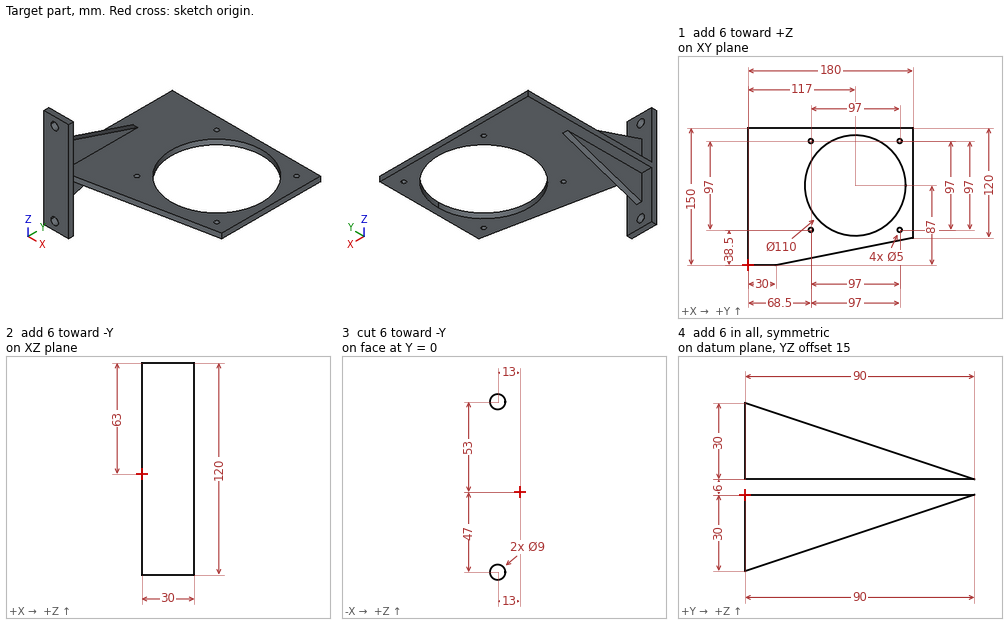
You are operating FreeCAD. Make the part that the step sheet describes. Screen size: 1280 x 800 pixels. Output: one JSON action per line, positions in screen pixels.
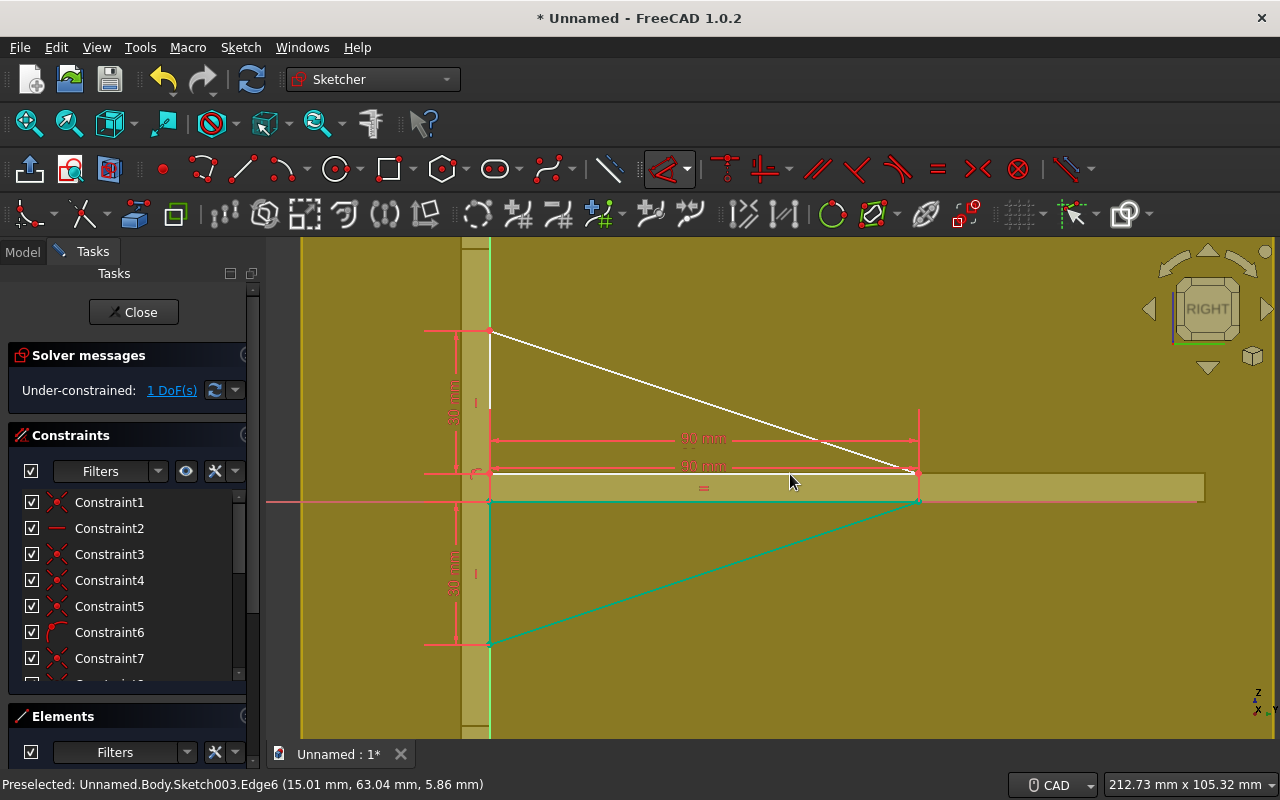
{"action": "scroll", "coordinate": [490, 474], "scroll_direction": "up", "scroll_amount": 2}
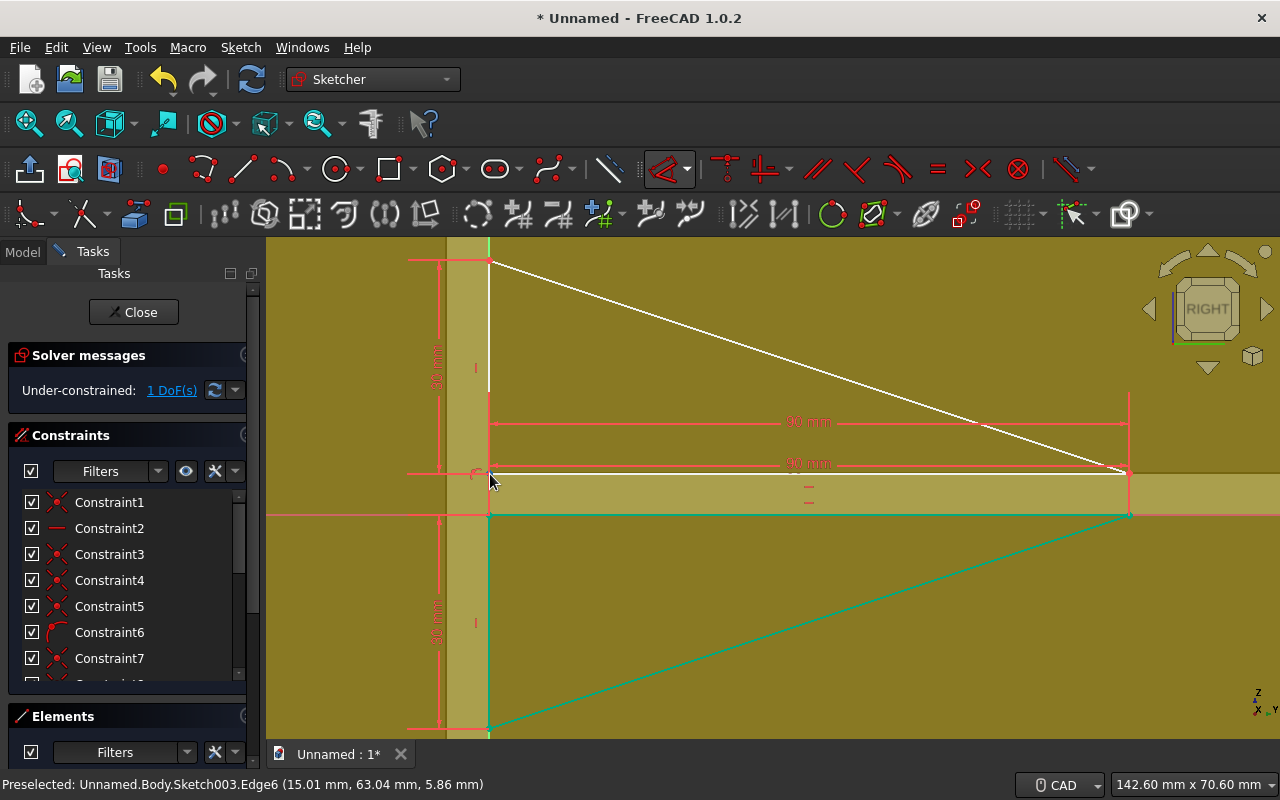
{"action": "left_click", "coordinate": [489, 474]}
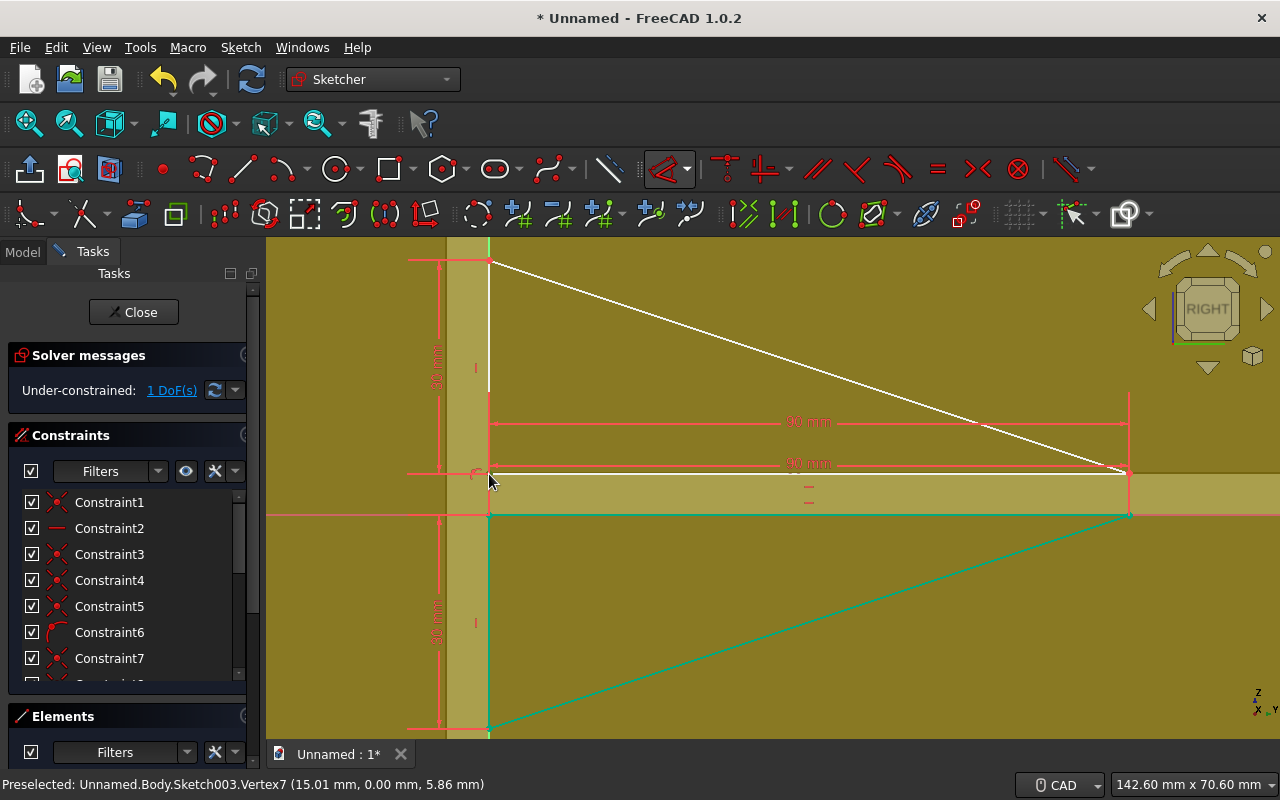
{"action": "key", "text": "i"}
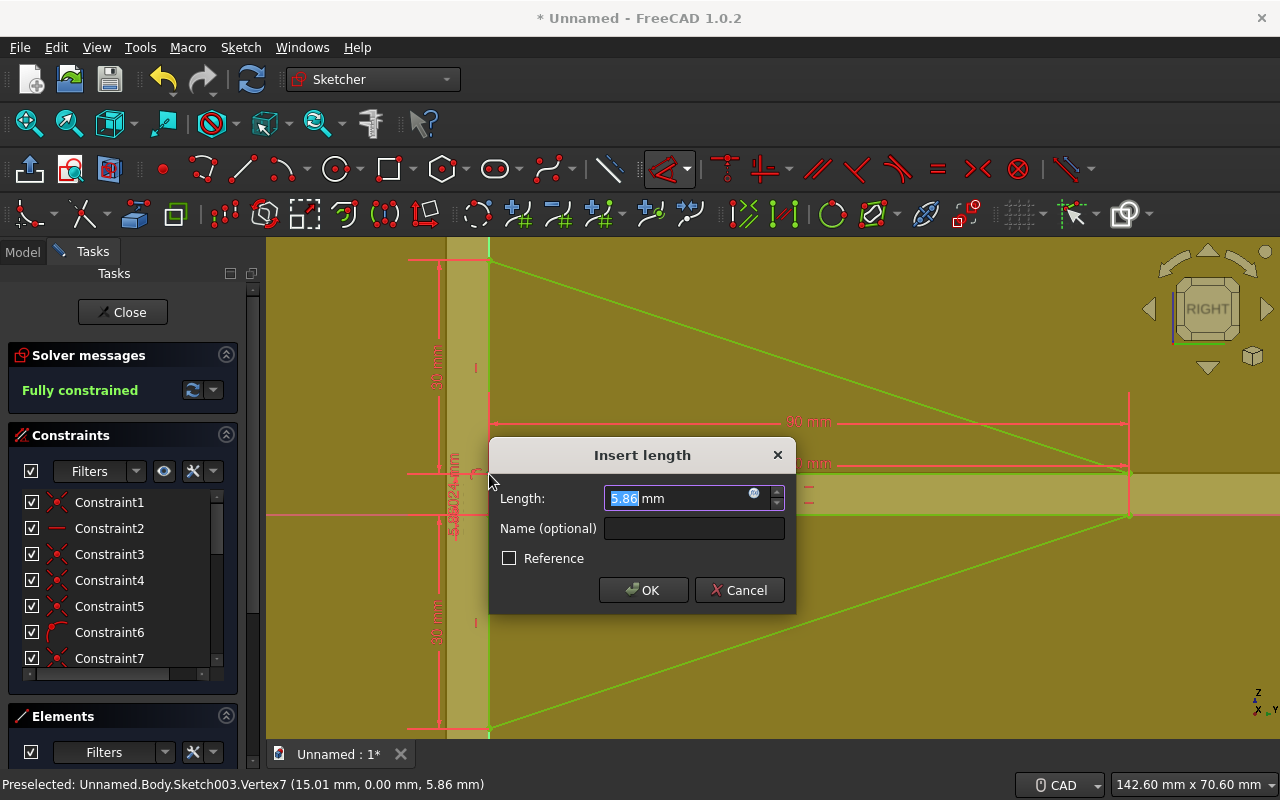
{"action": "type", "text": "6"}
{"action": "key", "text": "Return"}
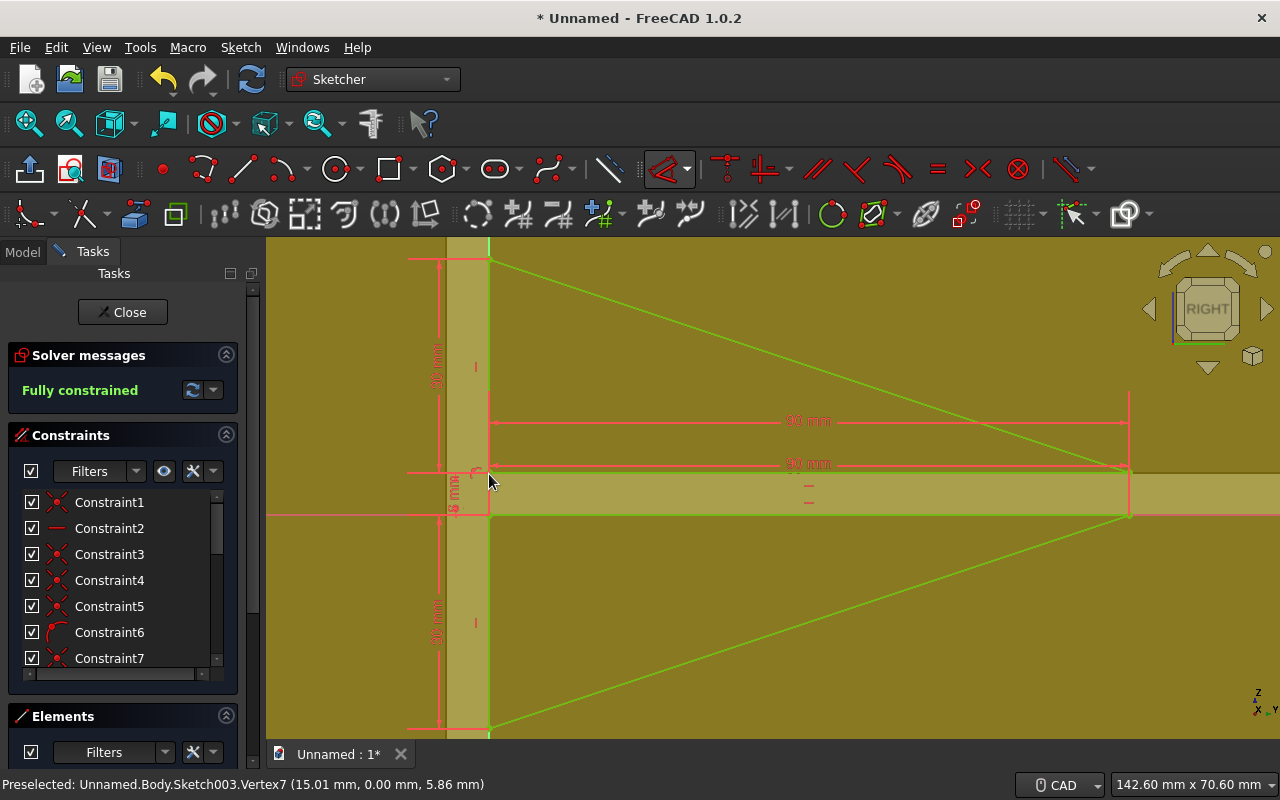
{"action": "left_click", "coordinate": [123, 312]}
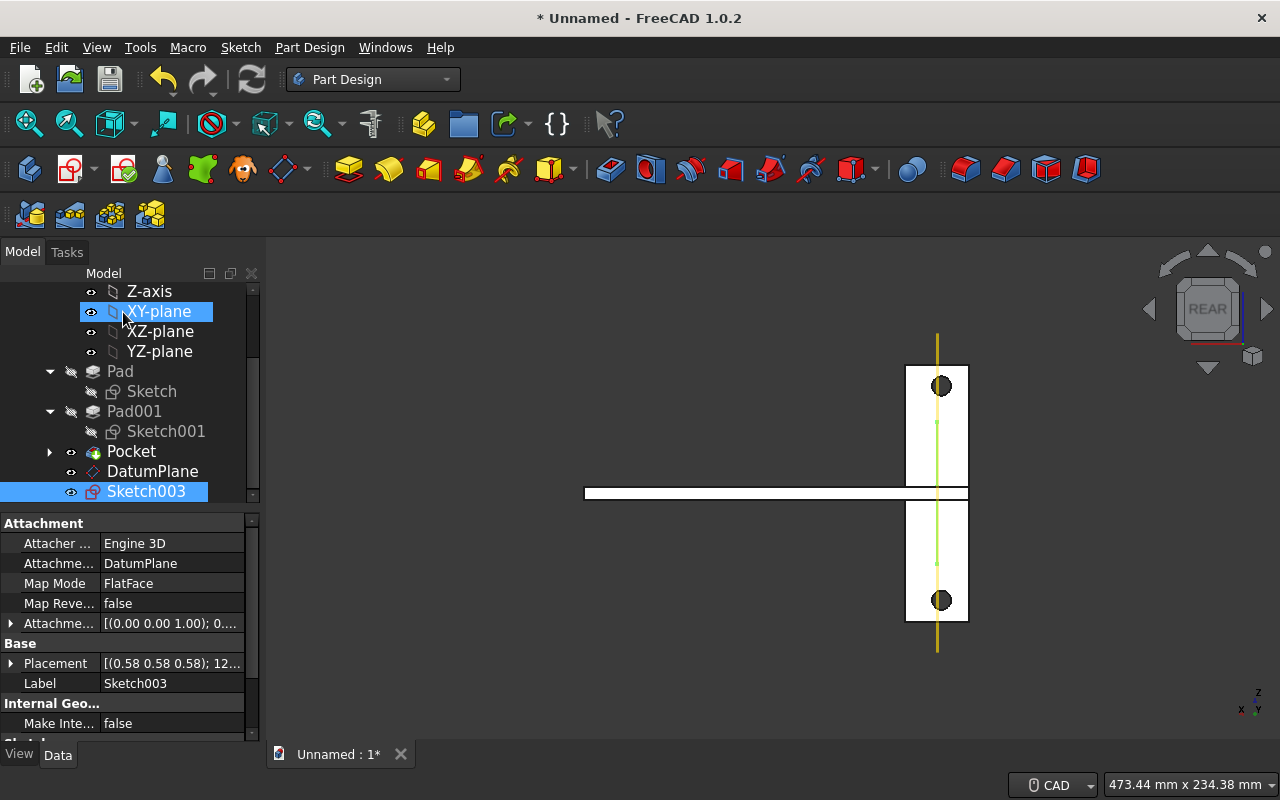
{"action": "left_click", "coordinate": [350, 170]}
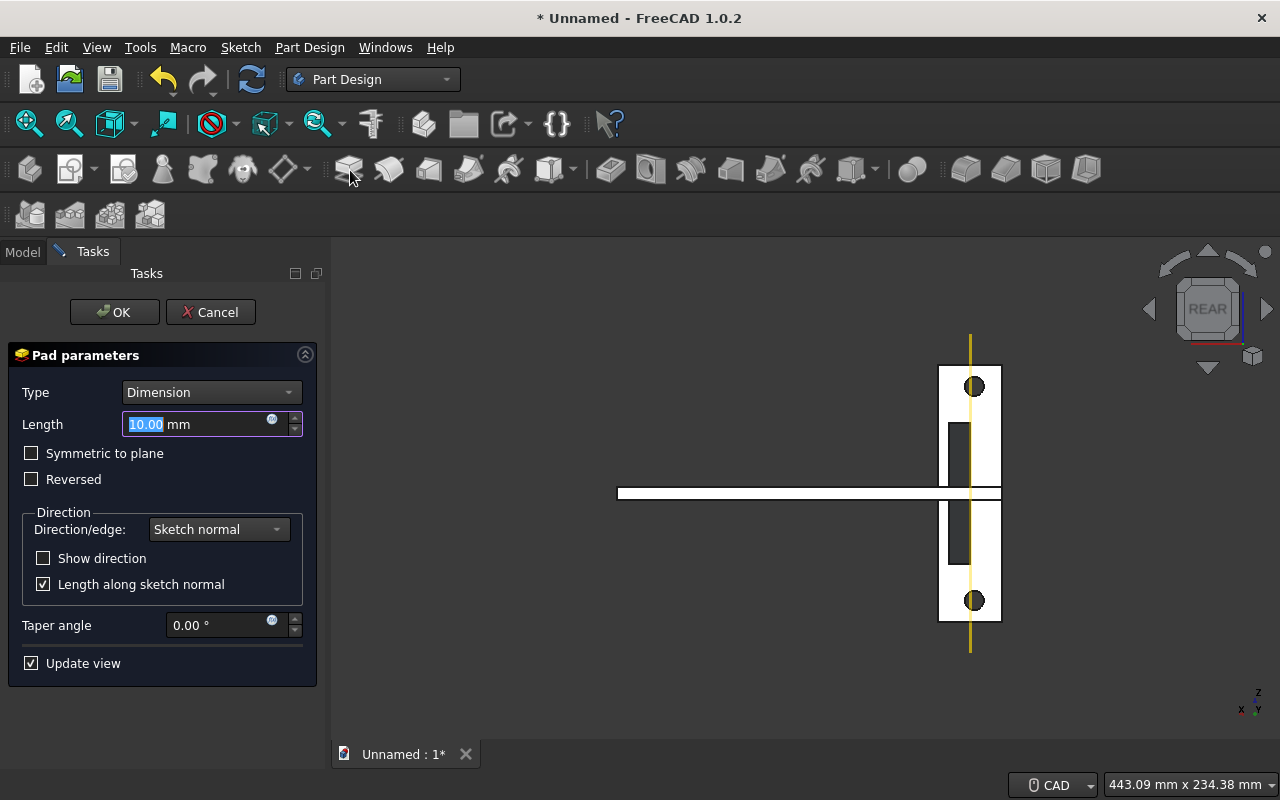
{"action": "type", "text": "6"}
{"action": "key", "text": "Tab"}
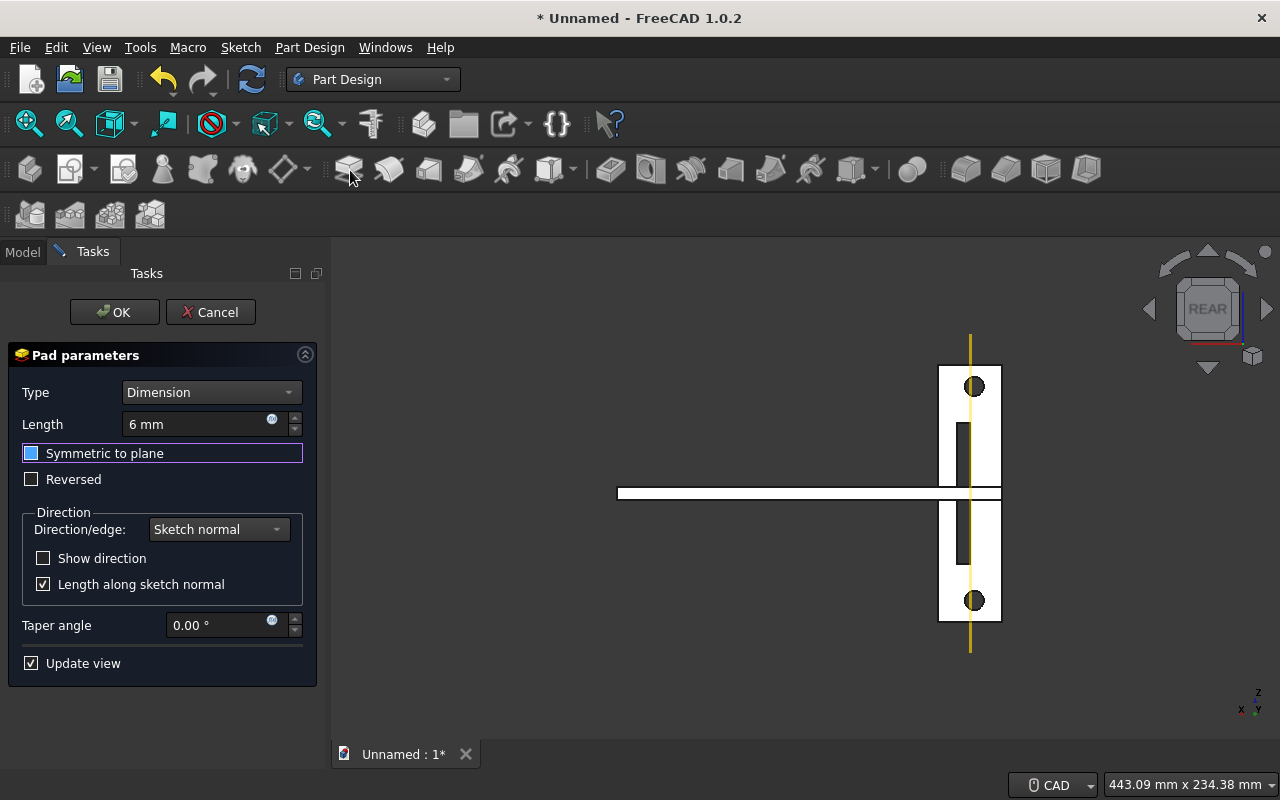
{"action": "left_click", "coordinate": [30, 453]}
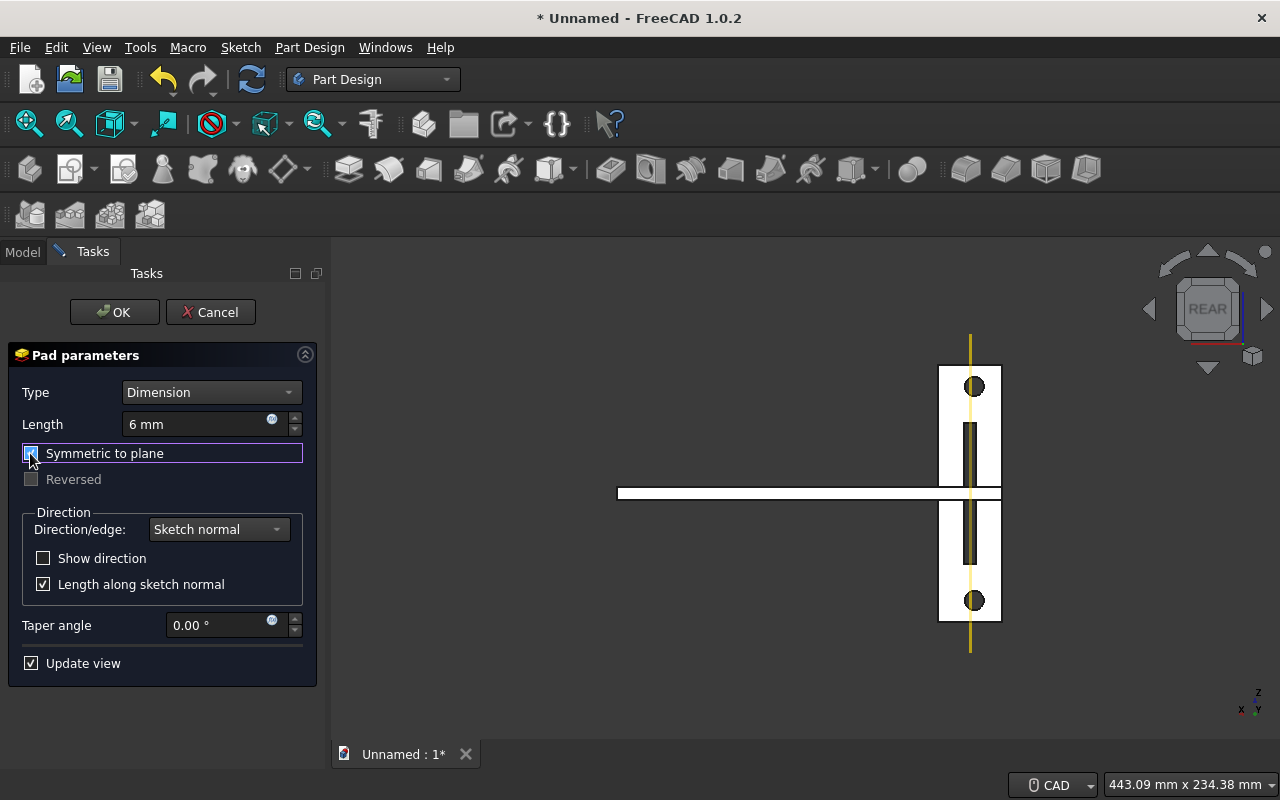
{"action": "left_click", "coordinate": [115, 312]}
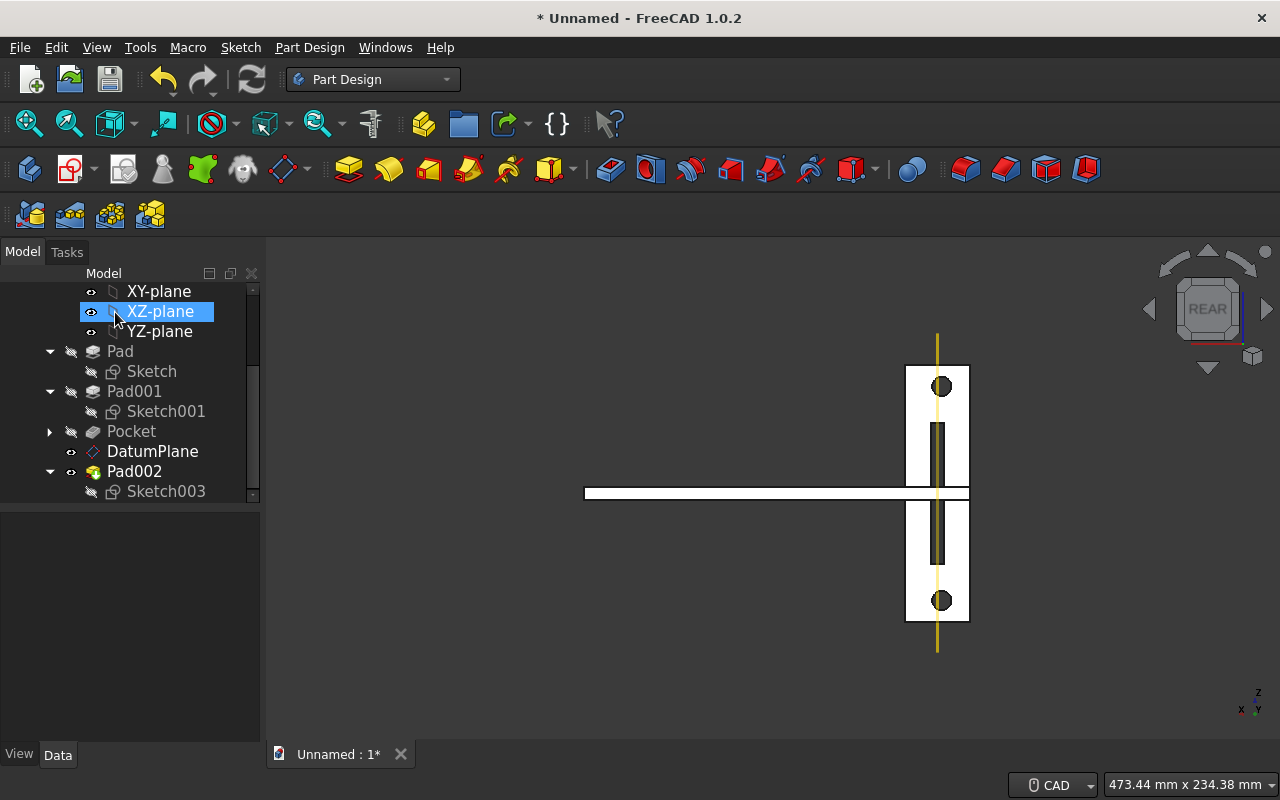
{"action": "left_click", "coordinate": [116, 452]}
{"action": "key", "text": "space"}